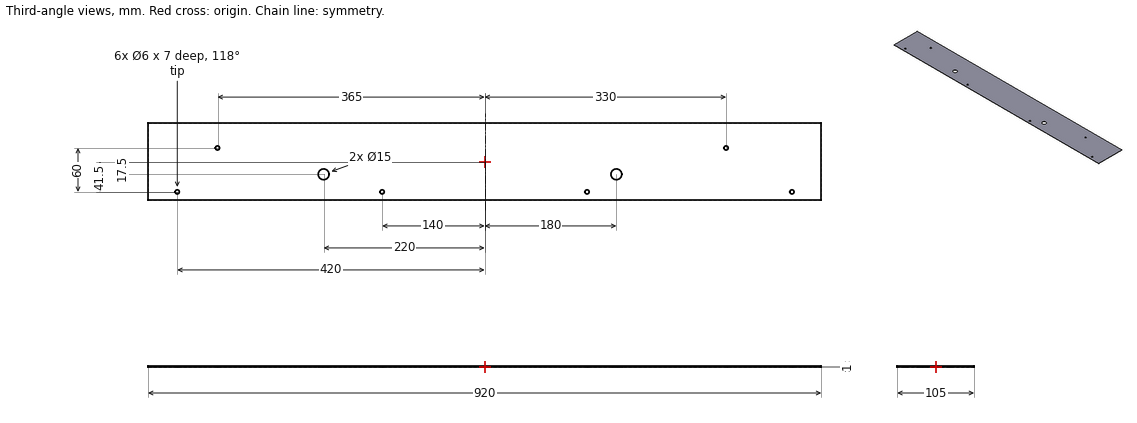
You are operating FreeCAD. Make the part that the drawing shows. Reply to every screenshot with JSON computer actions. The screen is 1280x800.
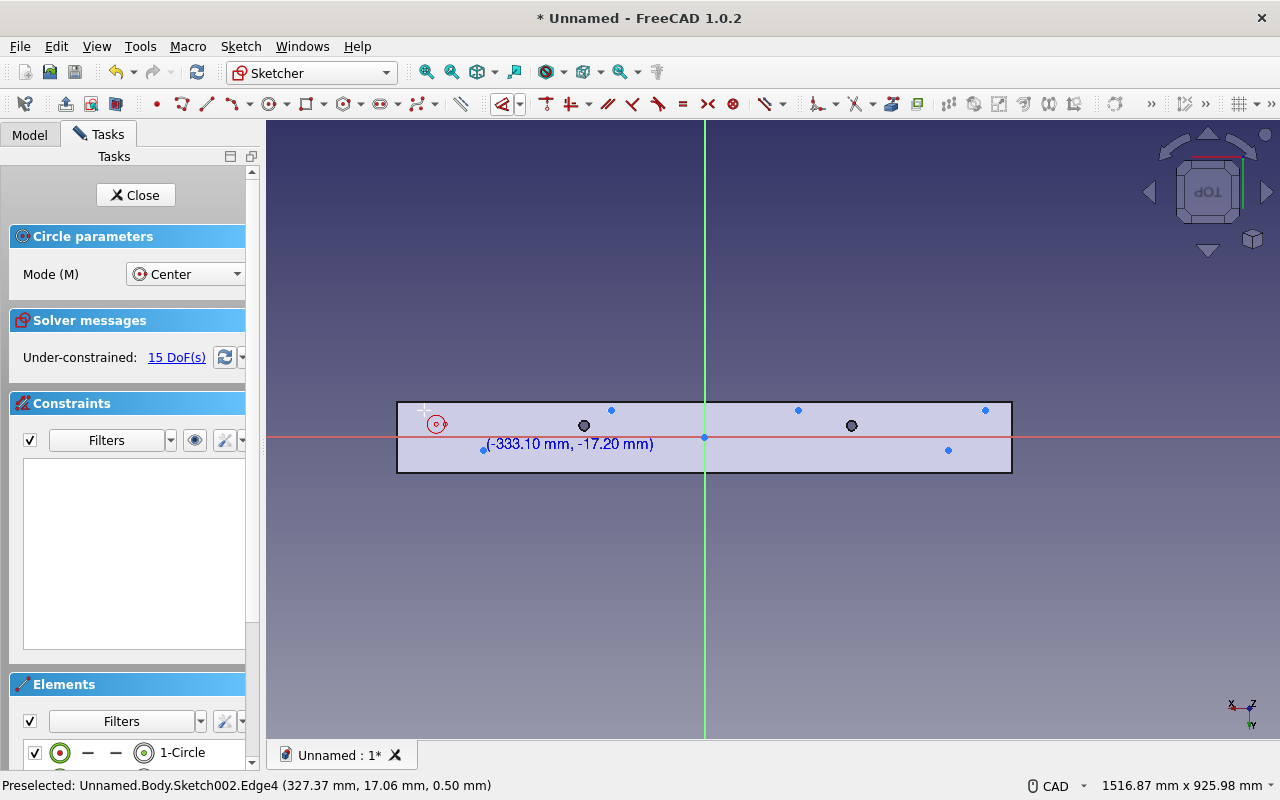
{"action": "left_click", "coordinate": [424, 410]}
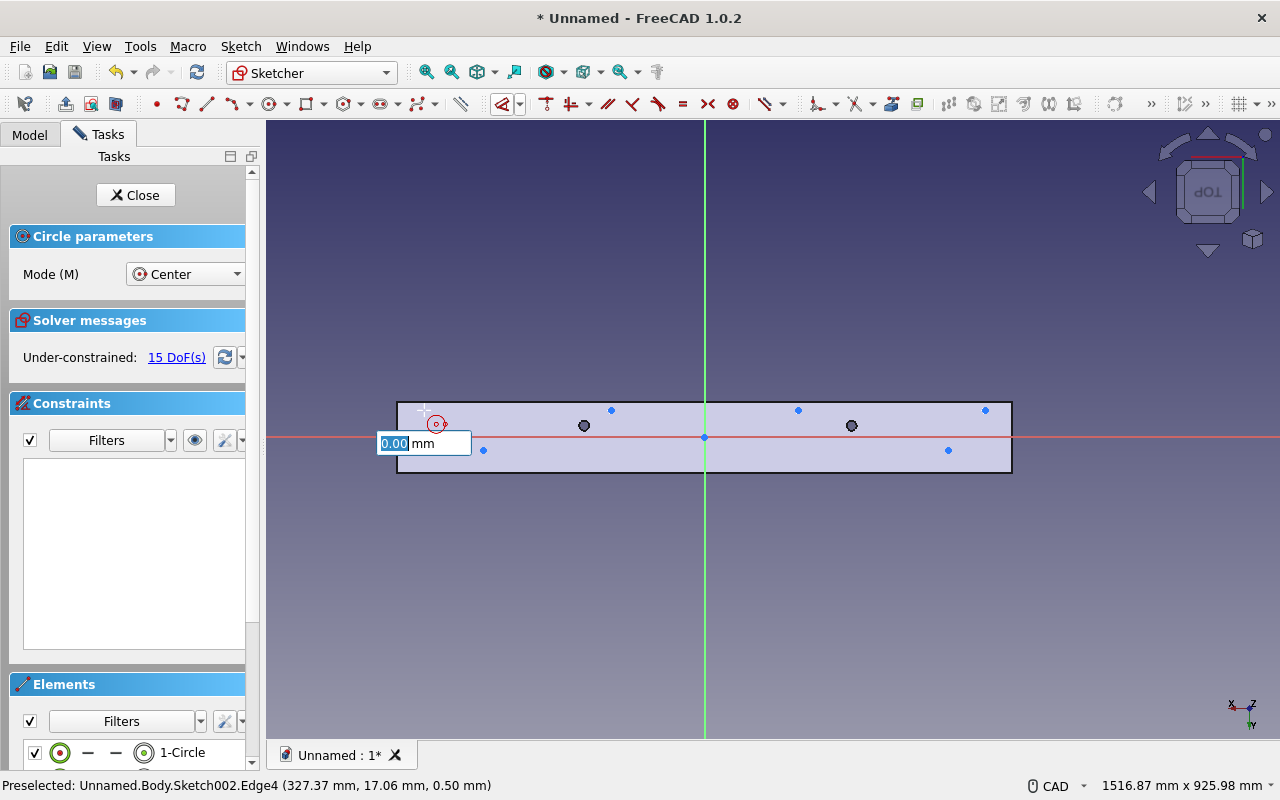
{"action": "scroll", "coordinate": [425, 408], "scroll_direction": "up", "scroll_amount": 11}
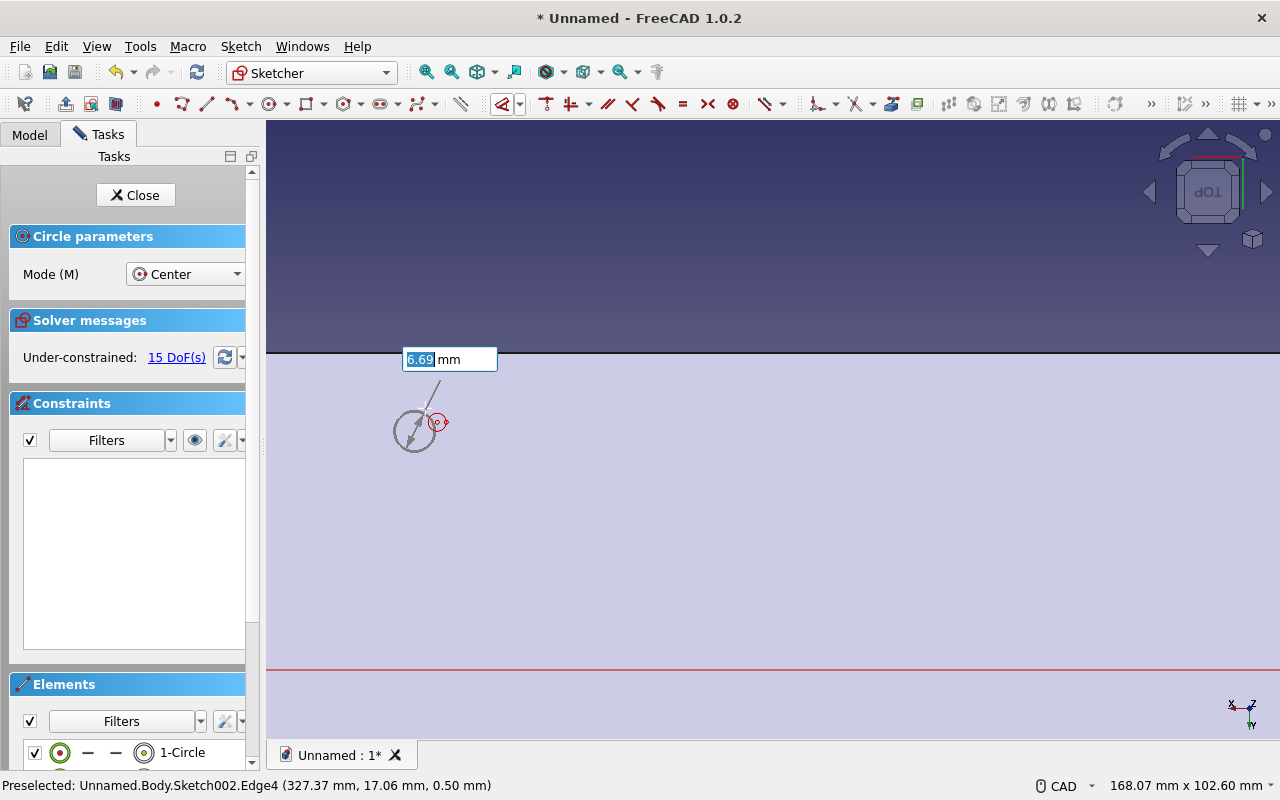
{"action": "left_click", "coordinate": [426, 407]}
{"action": "key", "text": "Escape"}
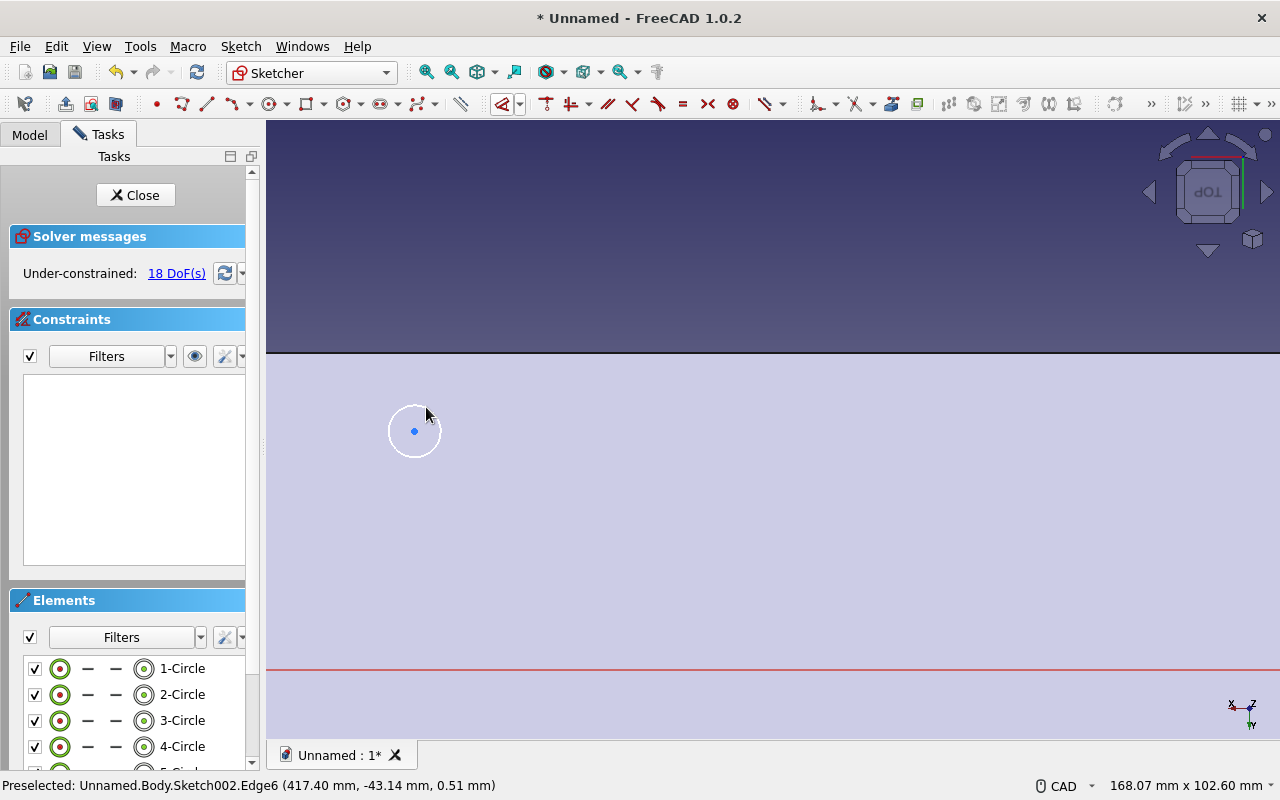
{"action": "scroll", "coordinate": [425, 408], "scroll_direction": "down", "scroll_amount": 11}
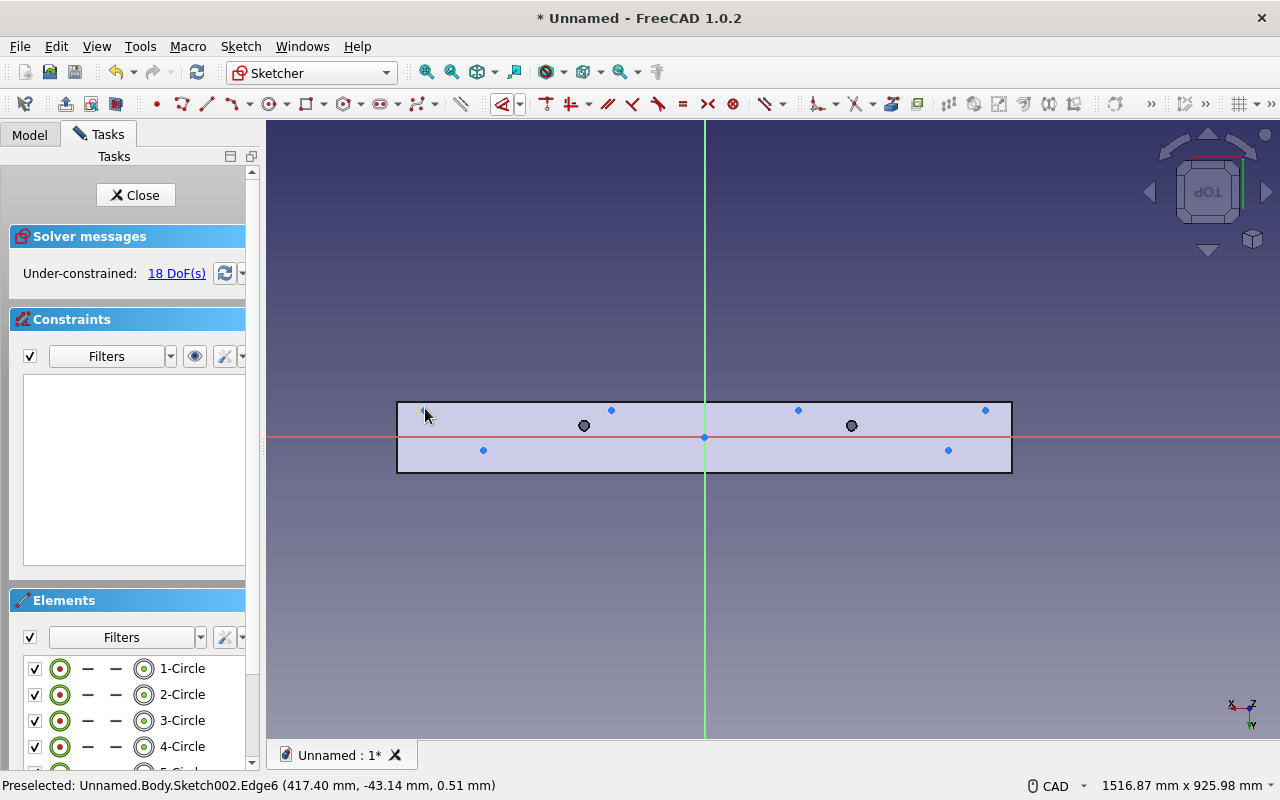
{"action": "scroll", "coordinate": [987, 409], "scroll_direction": "up", "scroll_amount": 9}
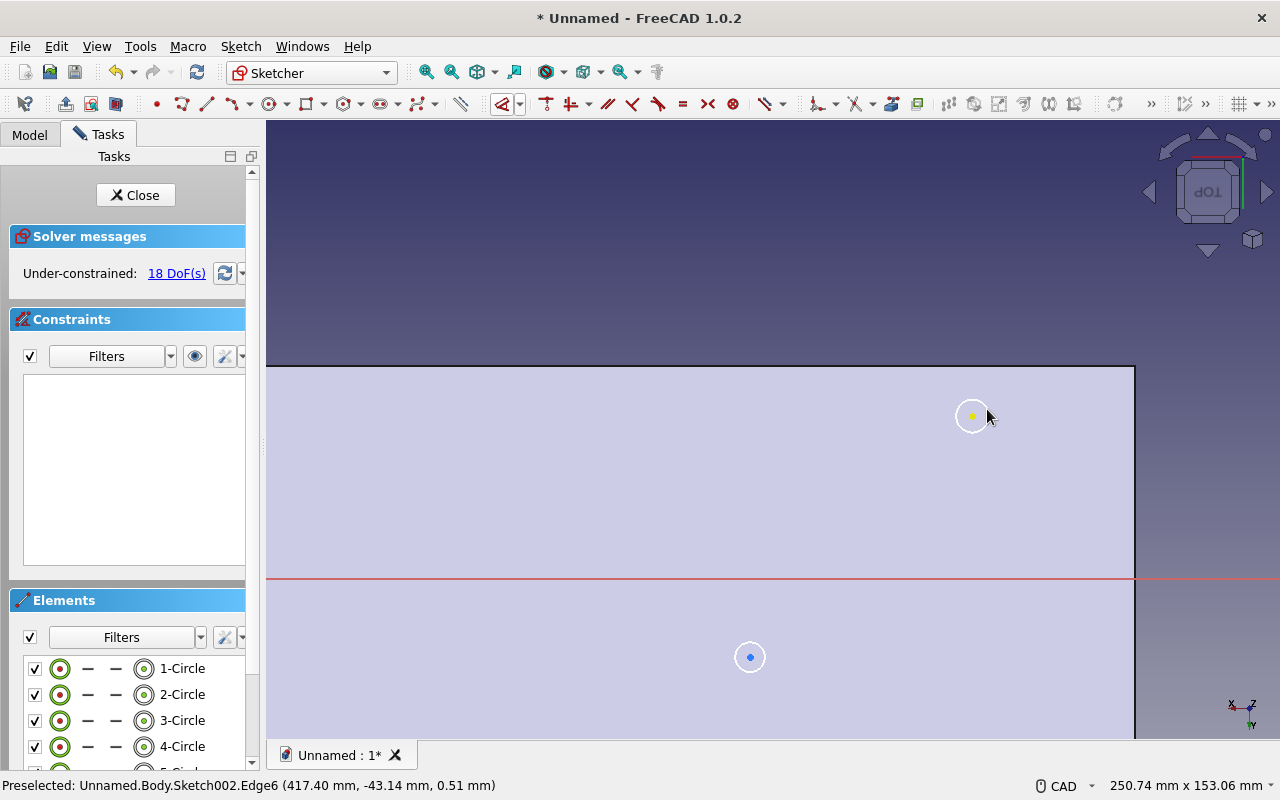
{"action": "left_click", "coordinate": [984, 404]}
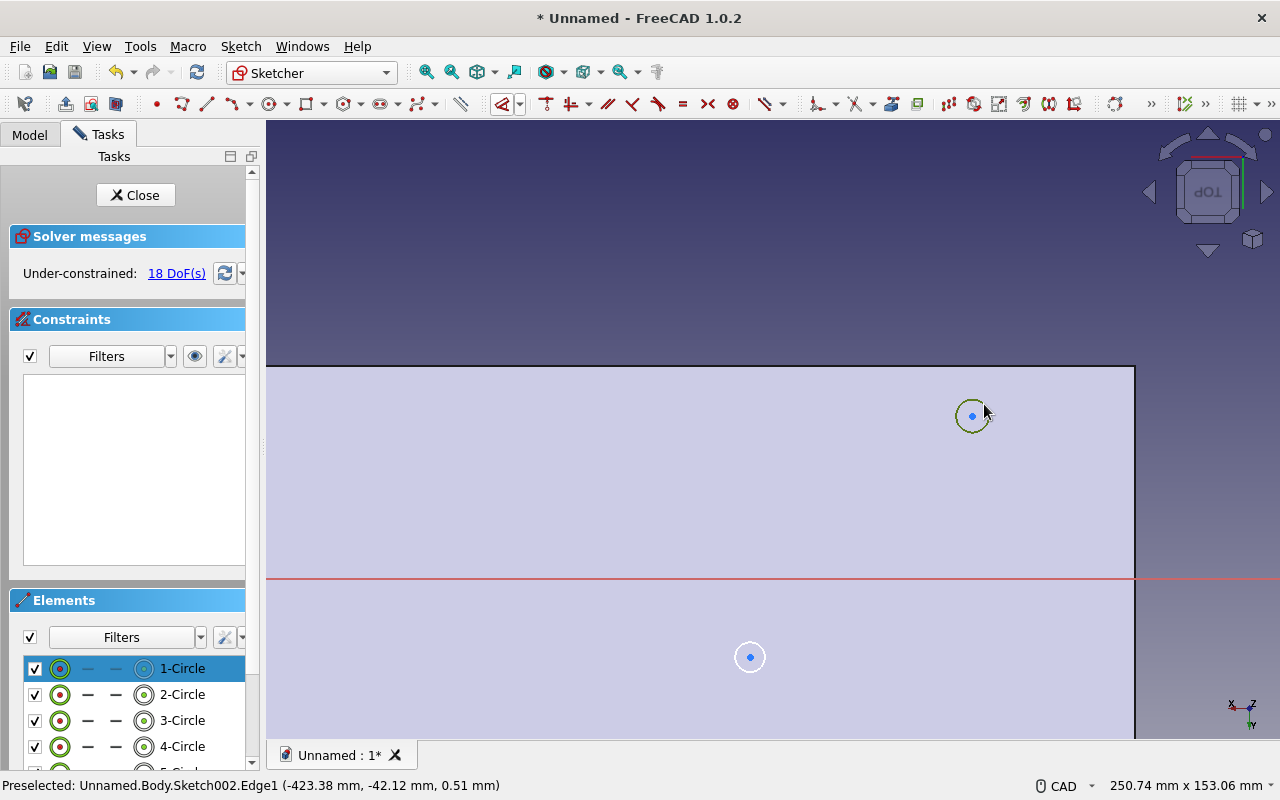
{"action": "scroll", "coordinate": [988, 409], "scroll_direction": "down", "scroll_amount": 9}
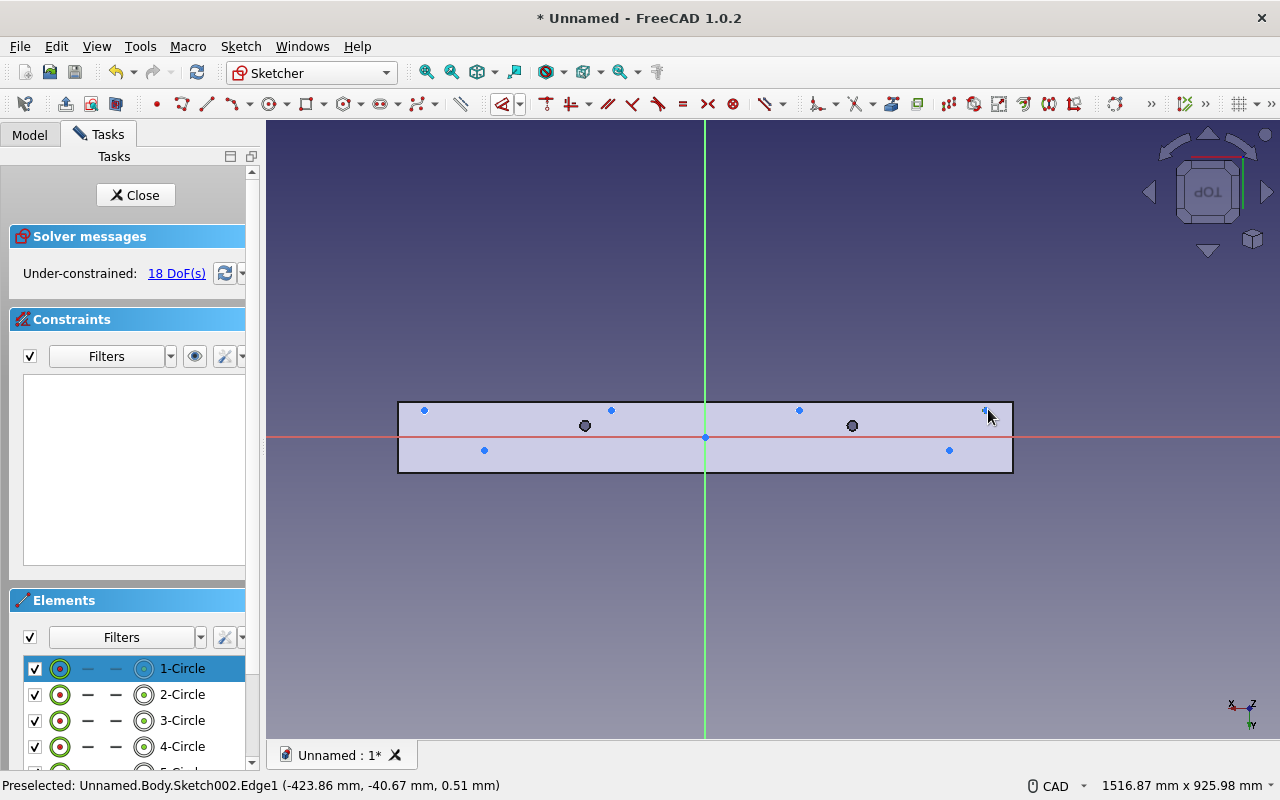
{"action": "scroll", "coordinate": [801, 409], "scroll_direction": "up", "scroll_amount": 9}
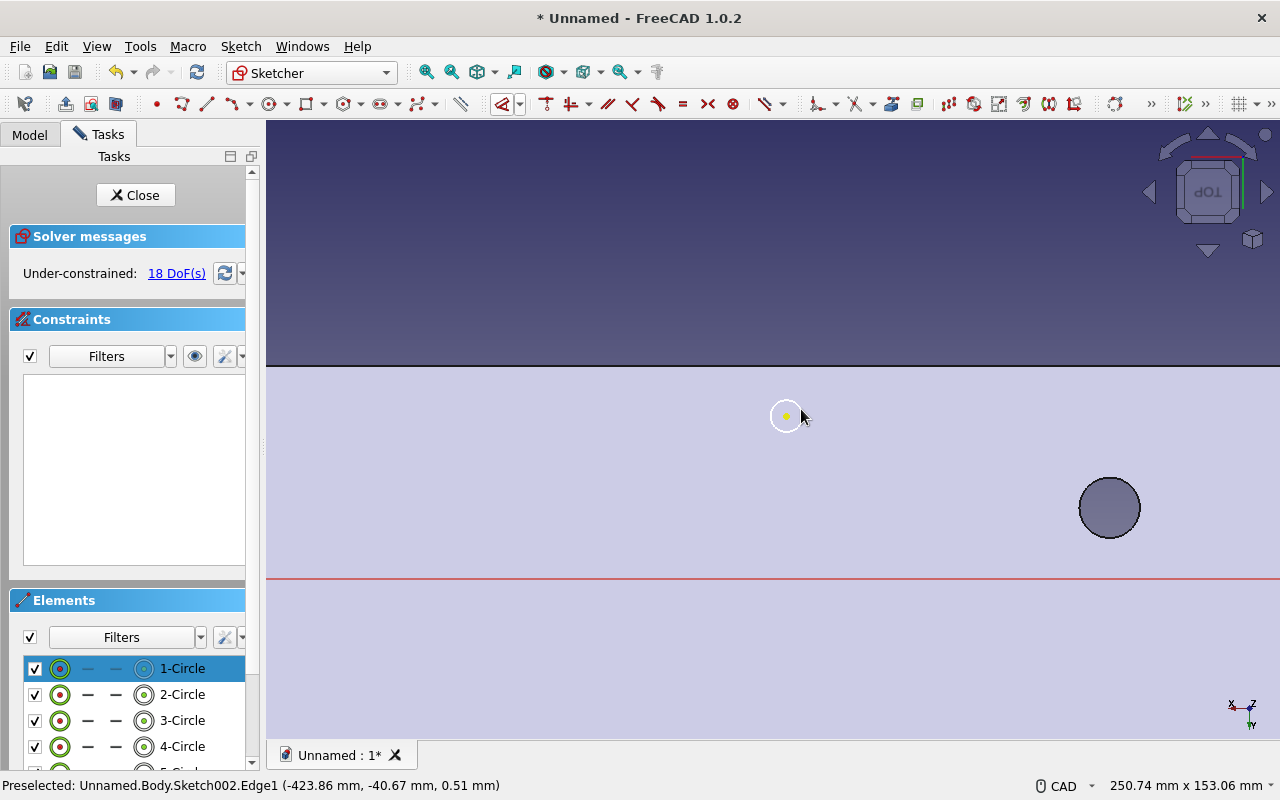
{"action": "left_click", "coordinate": [798, 405]}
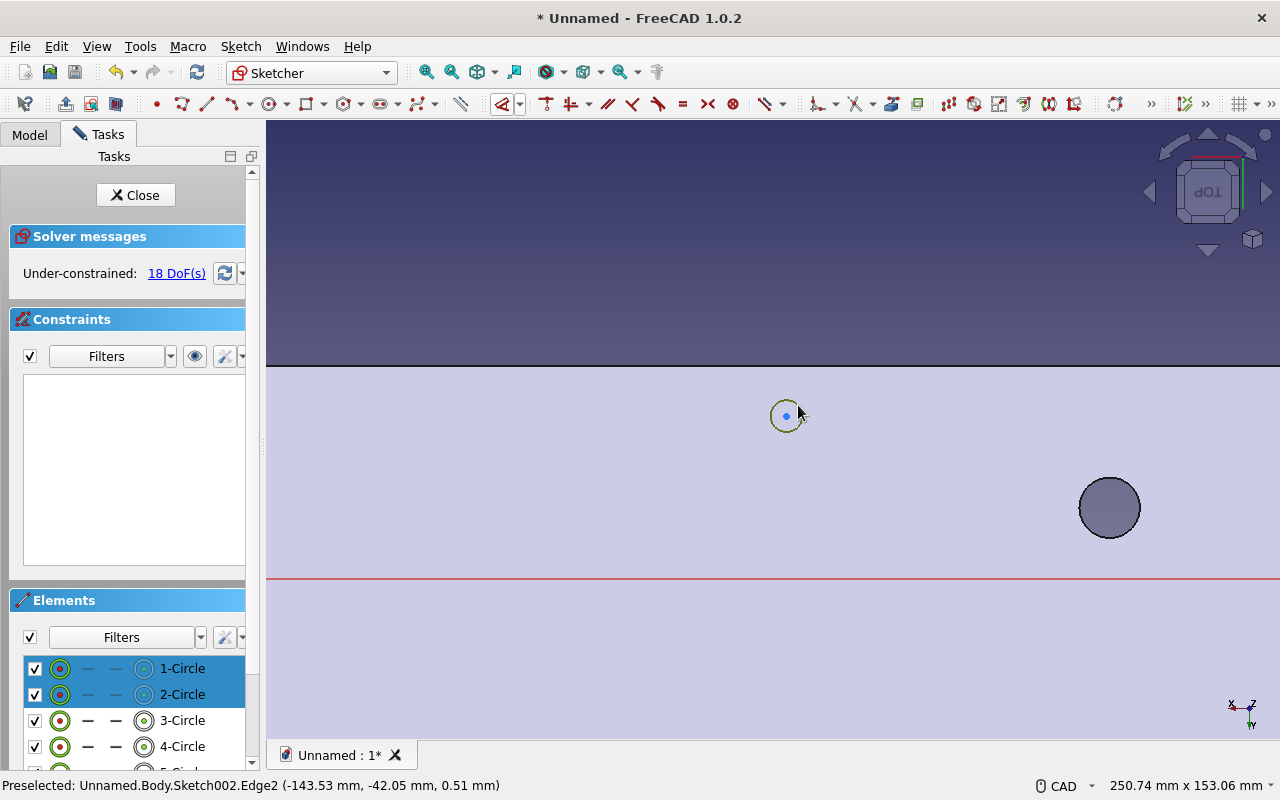
{"action": "scroll", "coordinate": [800, 409], "scroll_direction": "down", "scroll_amount": 9}